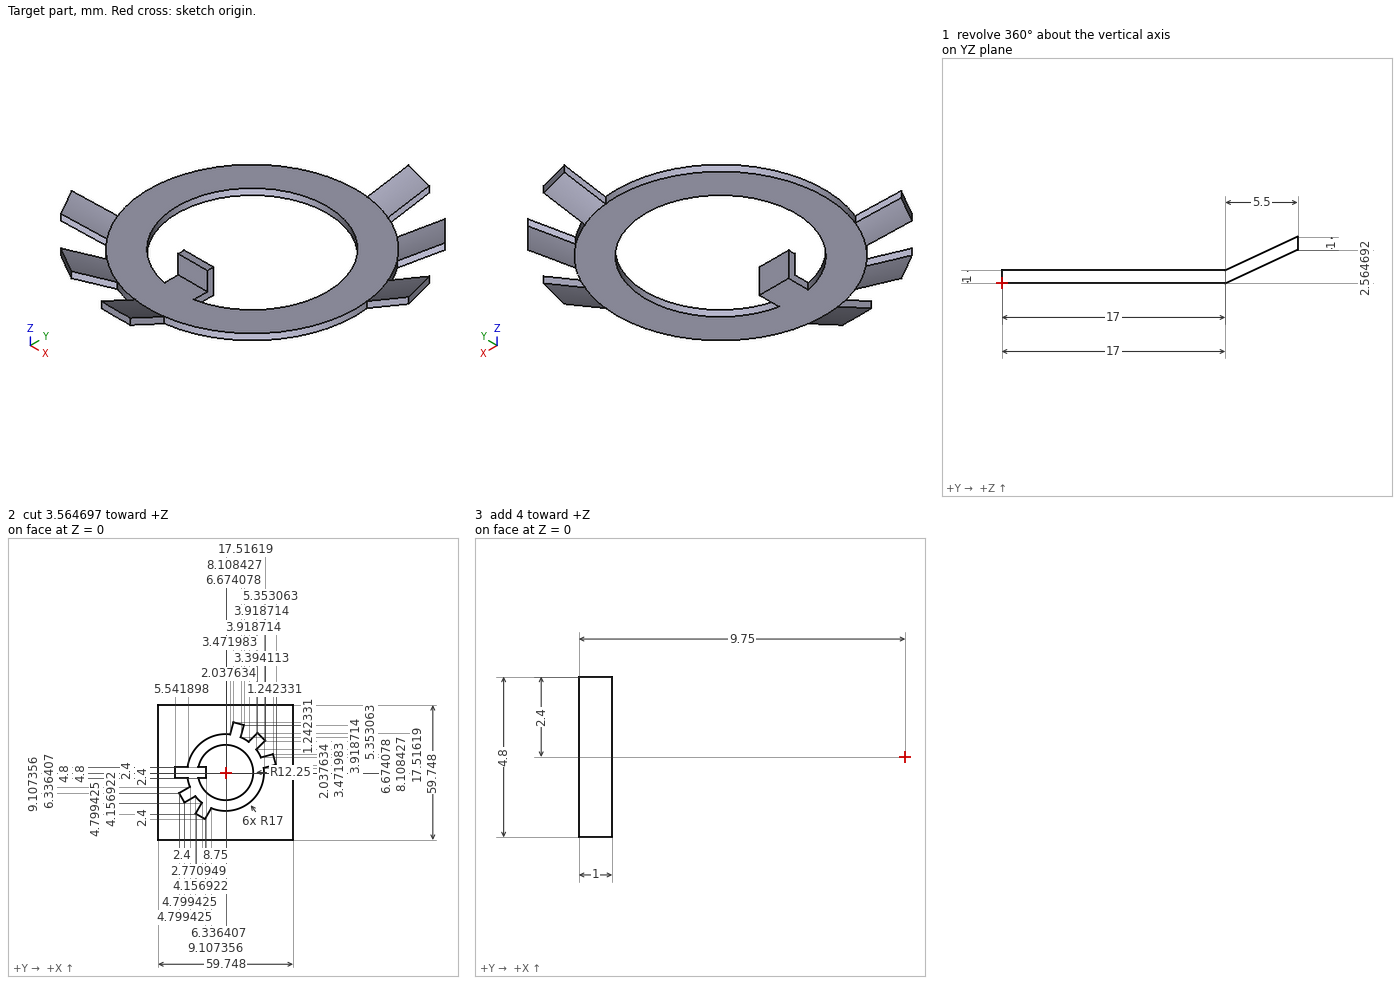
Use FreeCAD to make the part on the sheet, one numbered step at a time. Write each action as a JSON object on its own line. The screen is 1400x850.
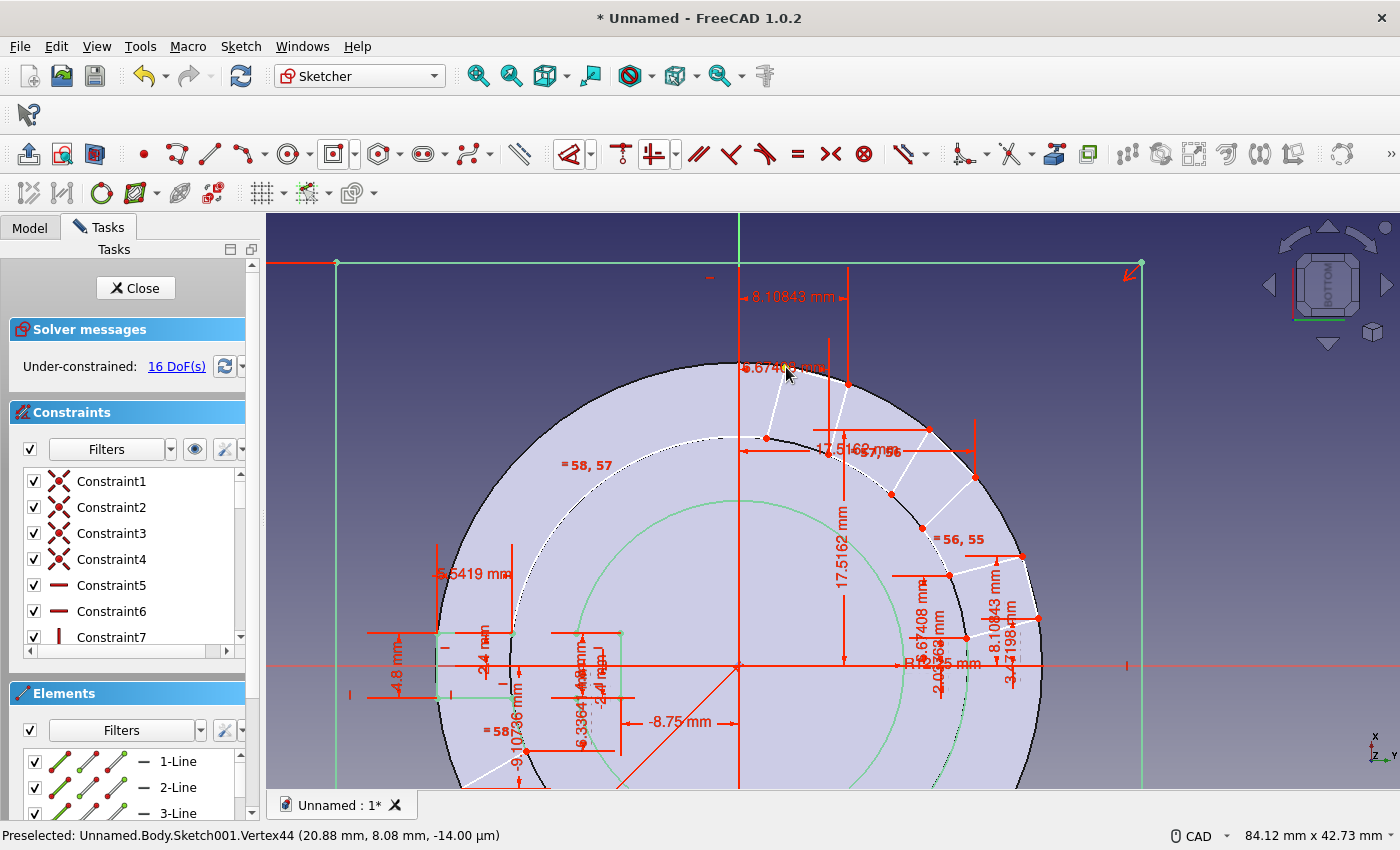
{"action": "left_click", "coordinate": [786, 367]}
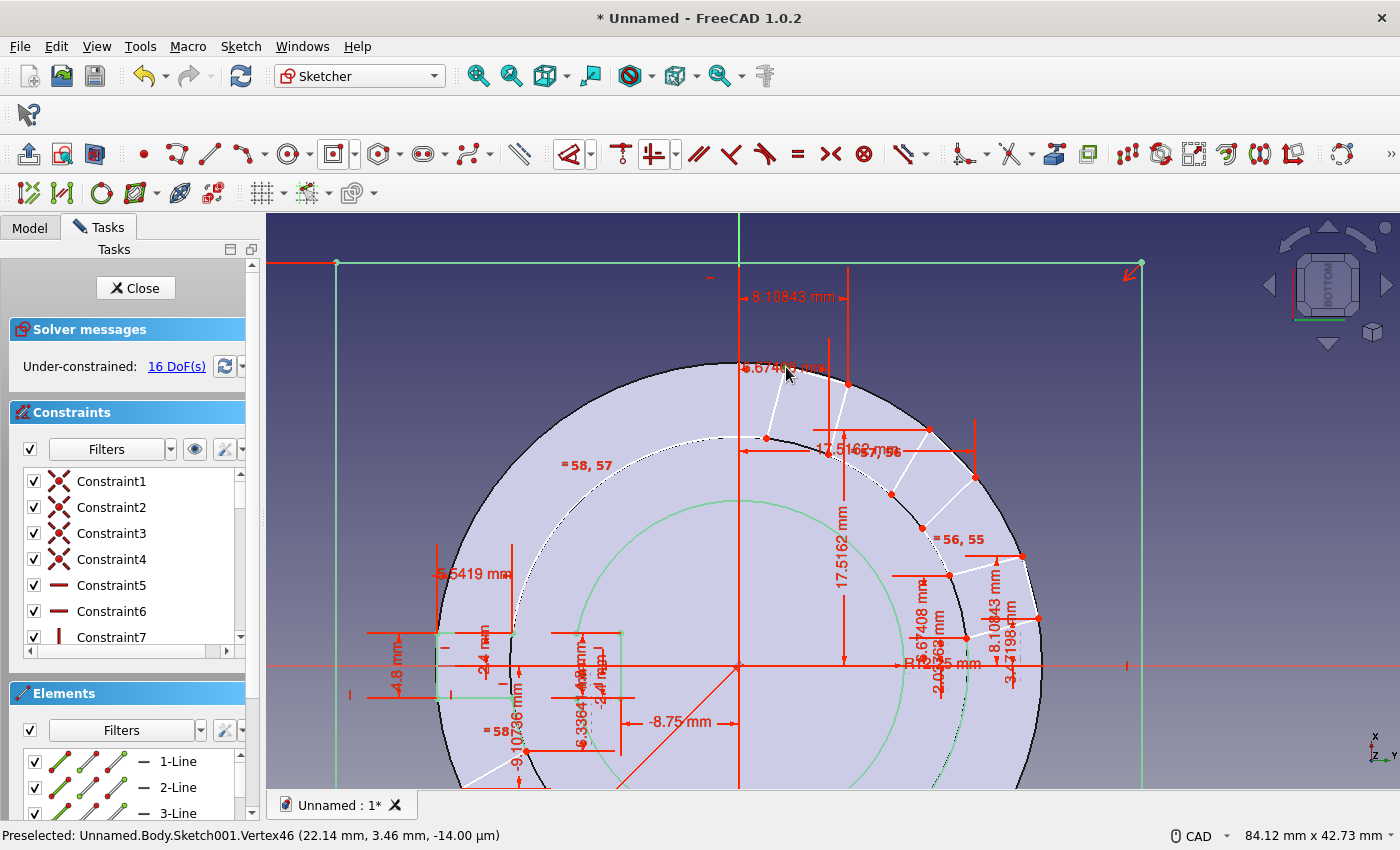
{"action": "key", "text": "l"}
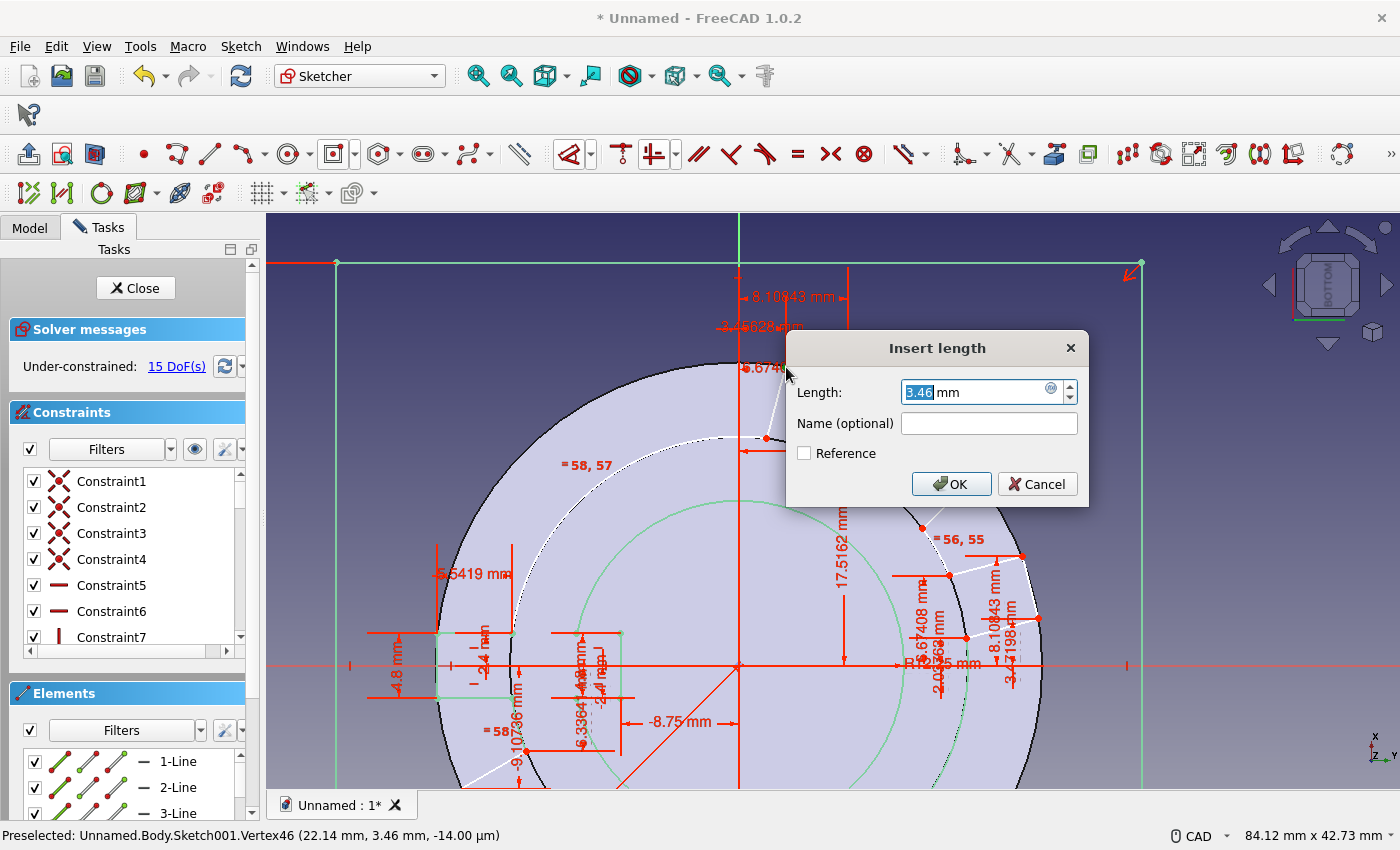
{"action": "type", "text": "3.471983"}
{"action": "key", "text": "Return"}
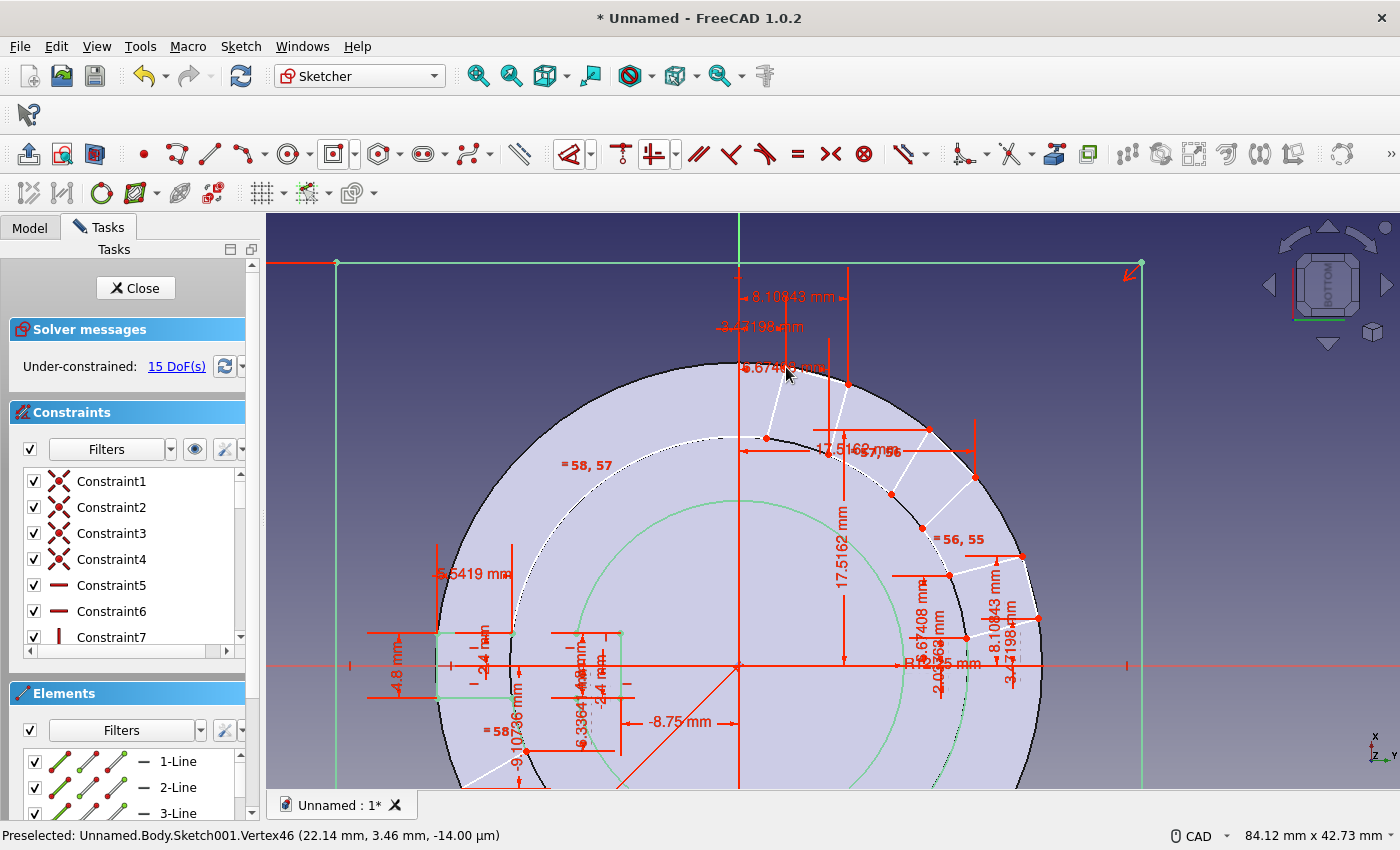
{"action": "scroll", "coordinate": [767, 438], "scroll_direction": "up", "scroll_amount": 2}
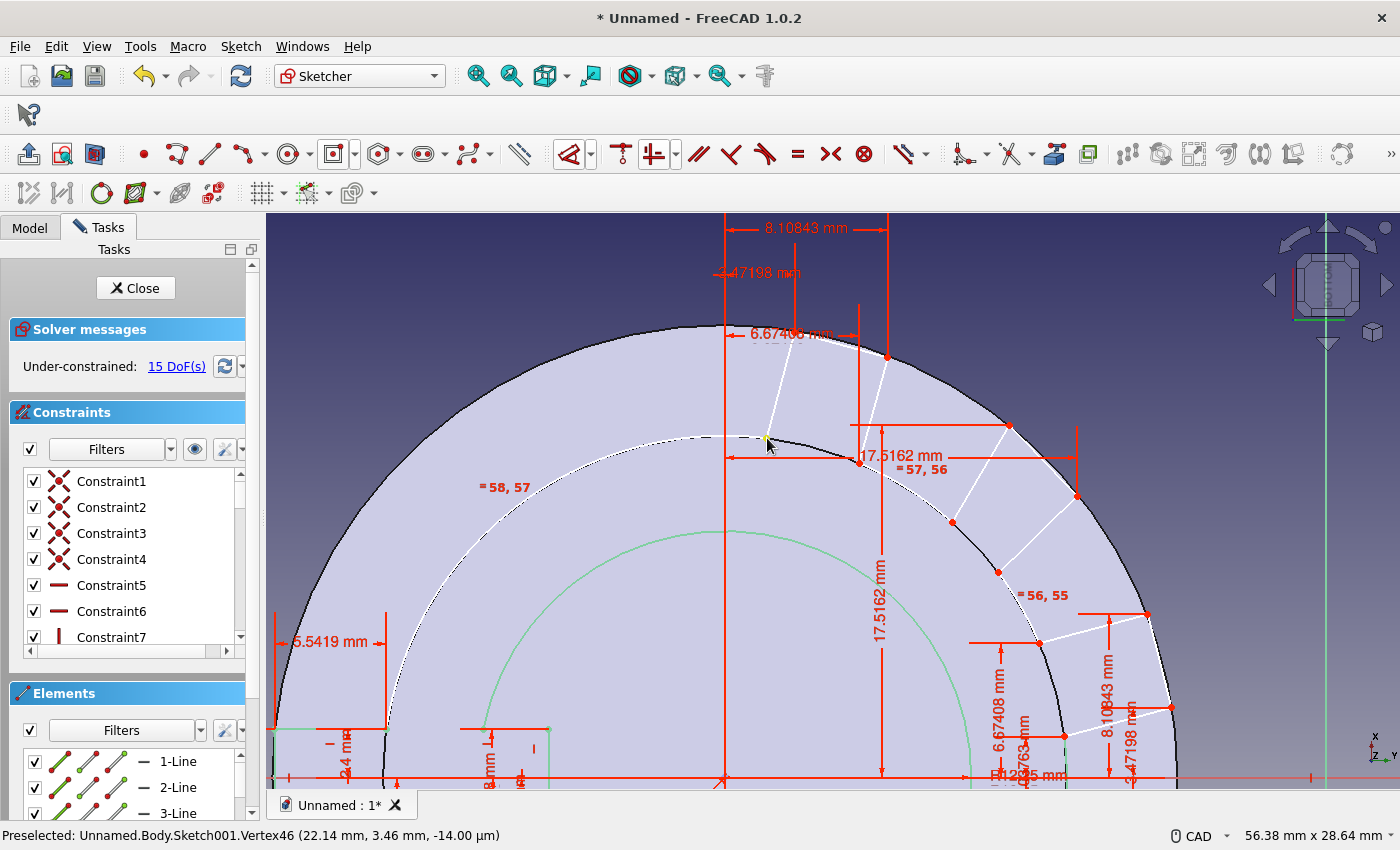
{"action": "left_click", "coordinate": [767, 438]}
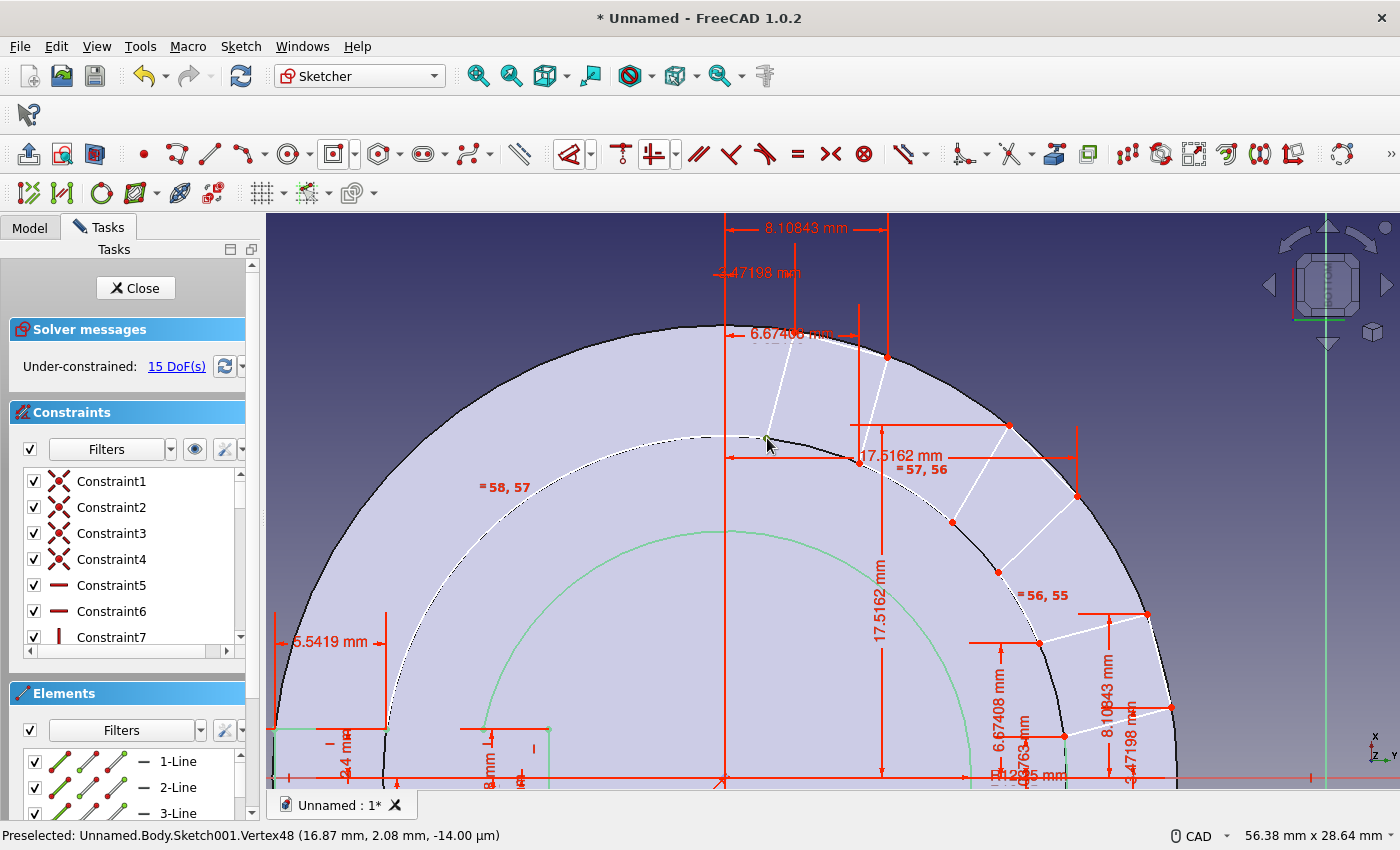
{"action": "left_click", "coordinate": [590, 154]}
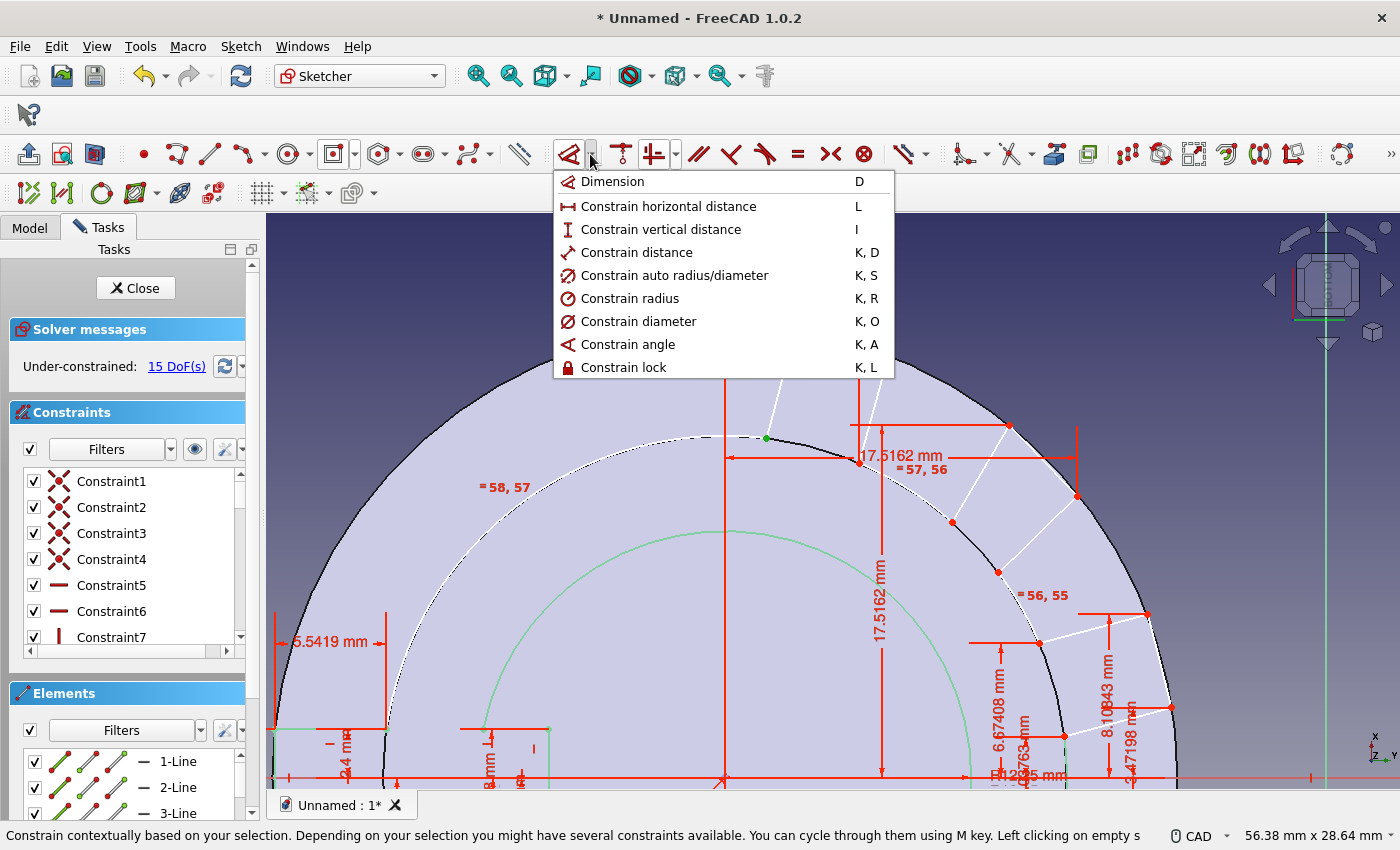
{"action": "left_click", "coordinate": [724, 206]}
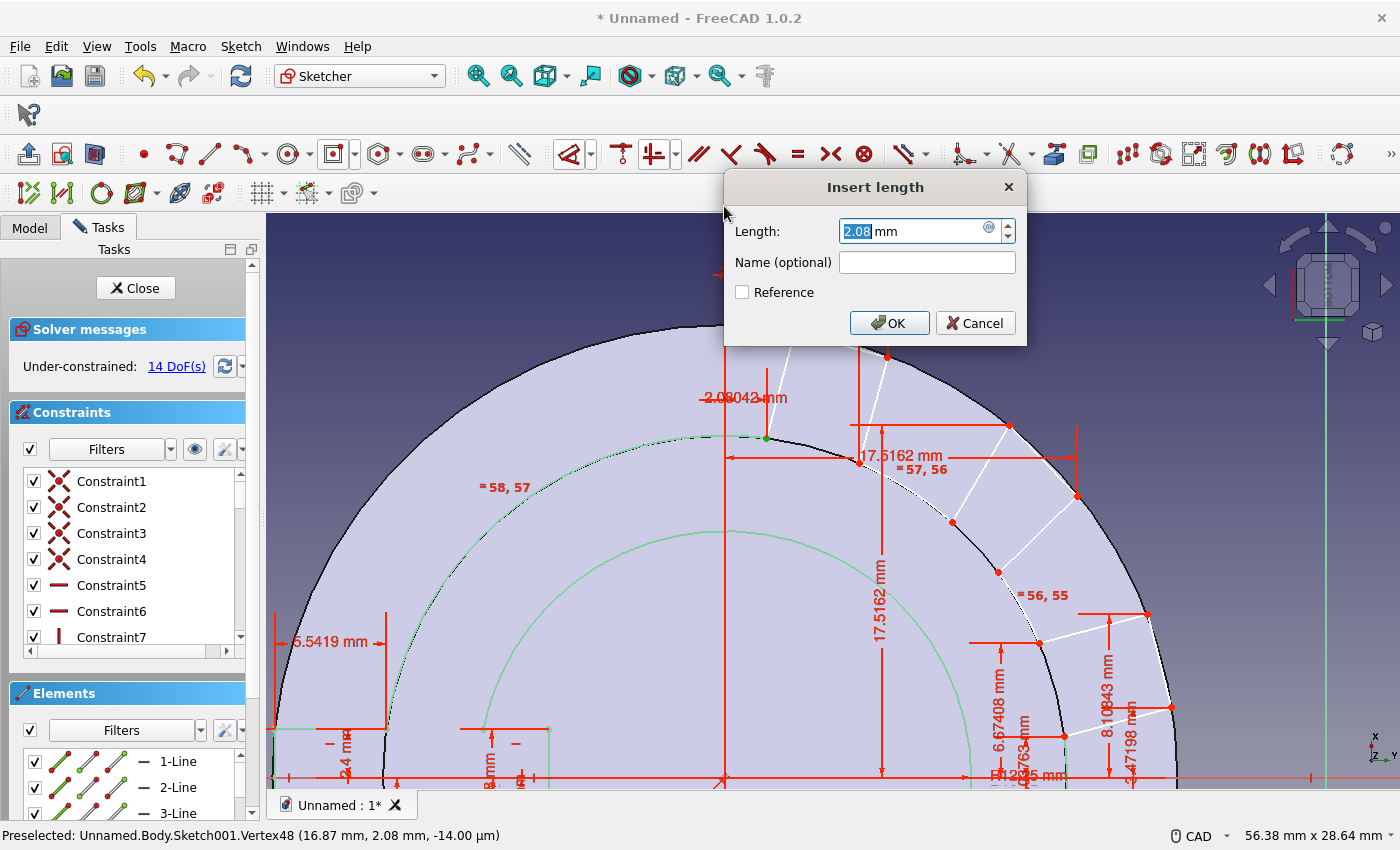
{"action": "type", "text": "2.037634"}
{"action": "key", "text": "Return"}